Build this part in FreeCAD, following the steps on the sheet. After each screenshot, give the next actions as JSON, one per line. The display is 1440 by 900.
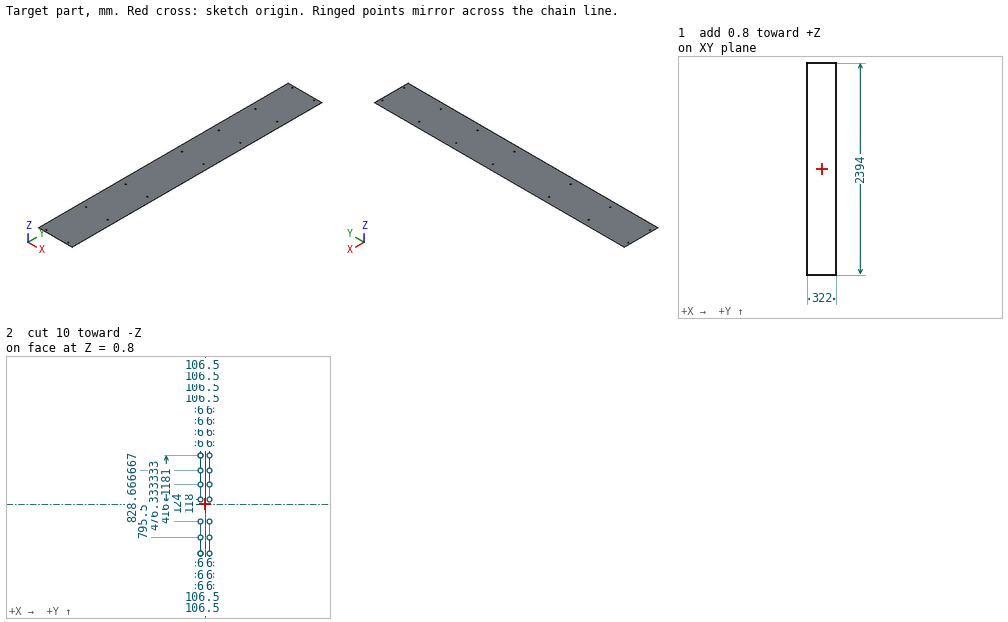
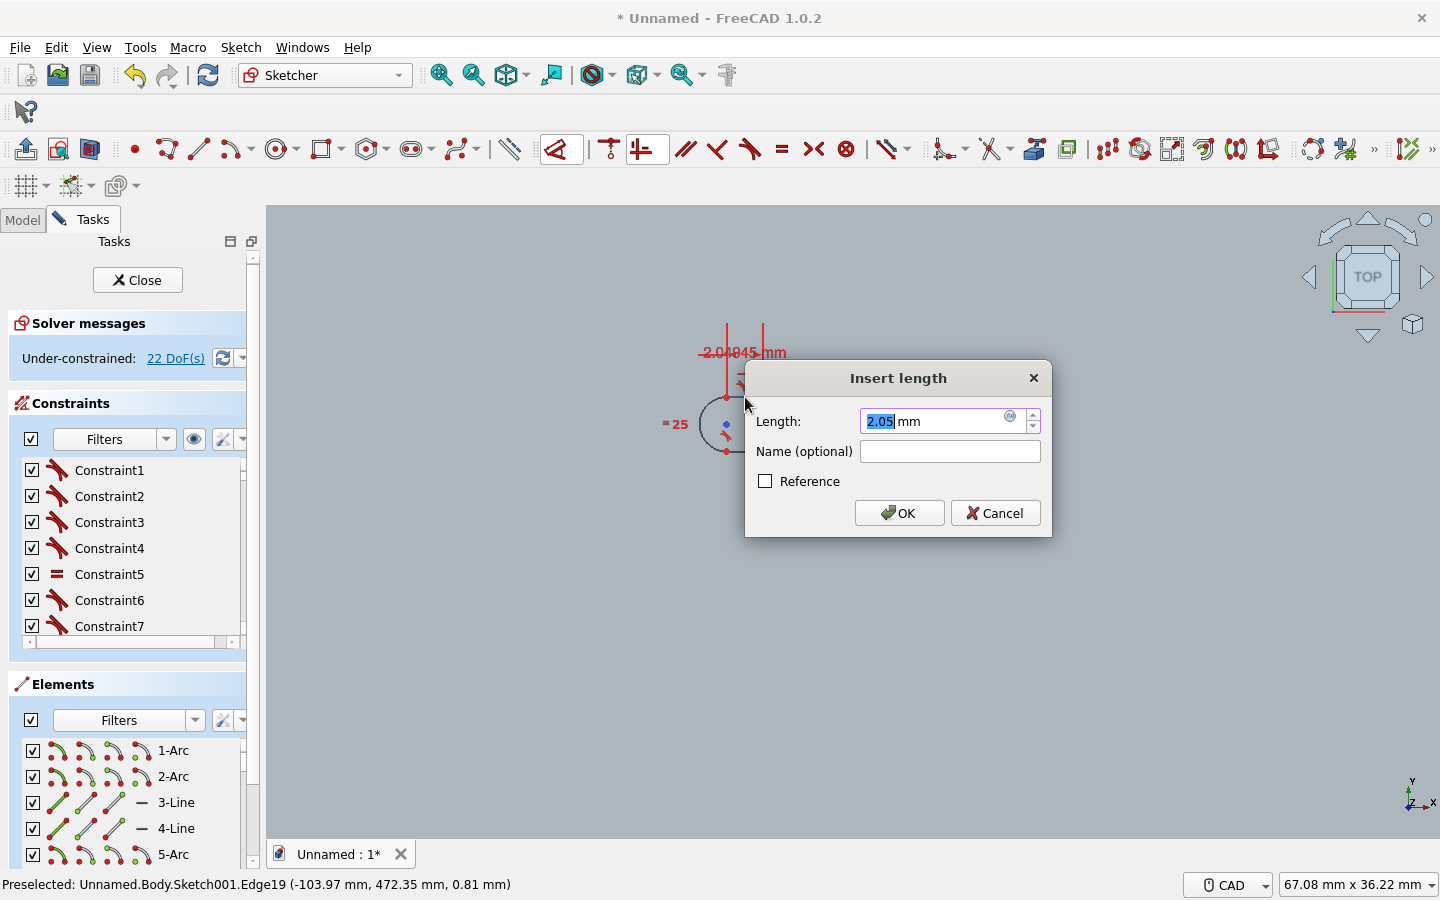
{"action": "type", "text": "6"}
{"action": "key", "text": "Return"}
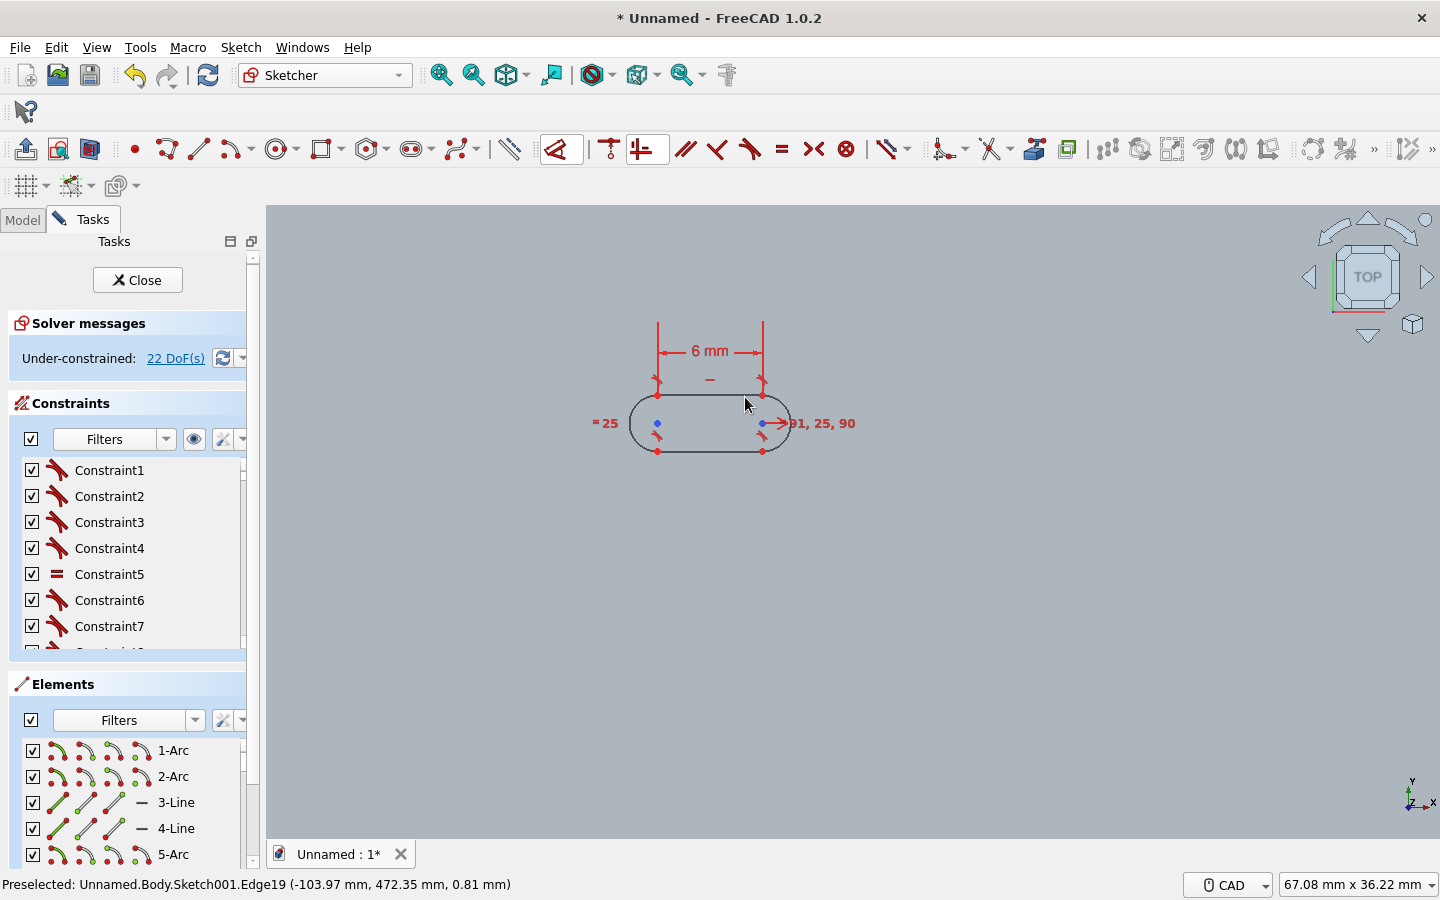
{"action": "scroll", "coordinate": [784, 522], "scroll_direction": "down", "scroll_amount": 15}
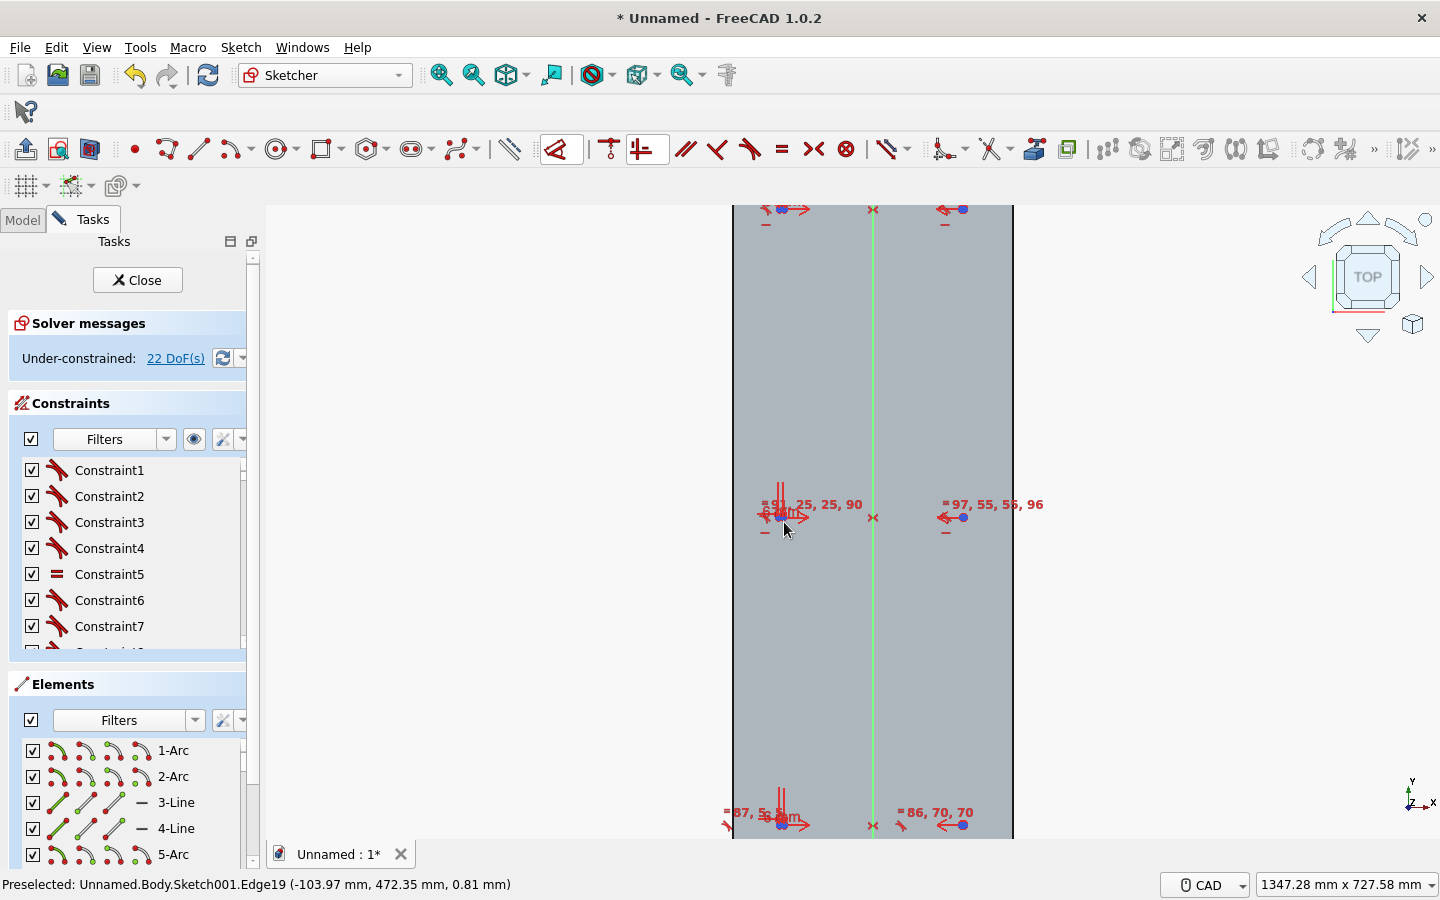
{"action": "scroll", "coordinate": [762, 419], "scroll_direction": "down", "scroll_amount": 8}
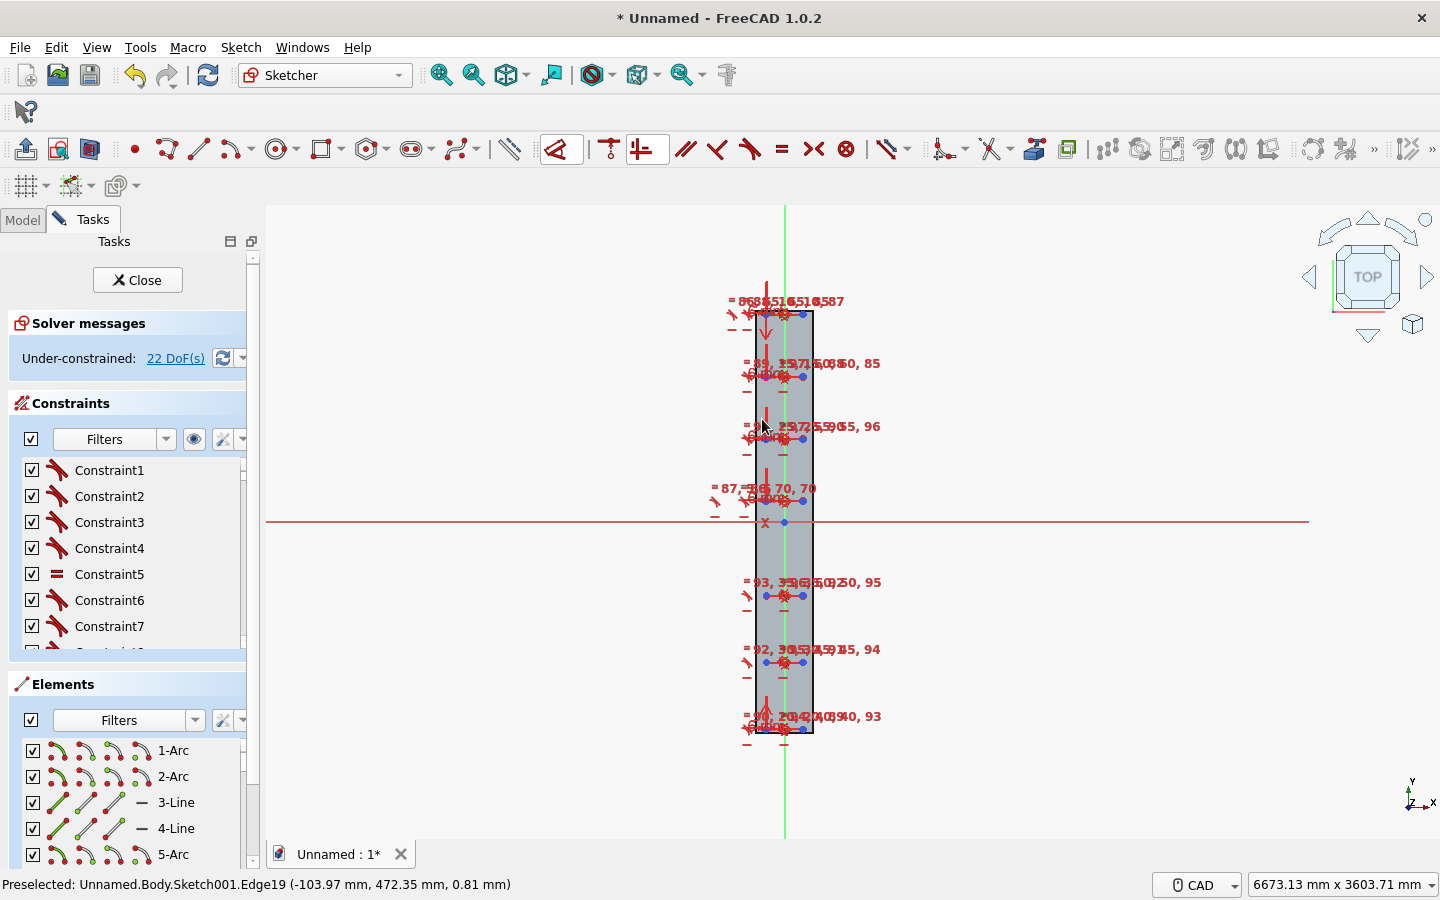
{"action": "scroll", "coordinate": [766, 662], "scroll_direction": "up", "scroll_amount": 19}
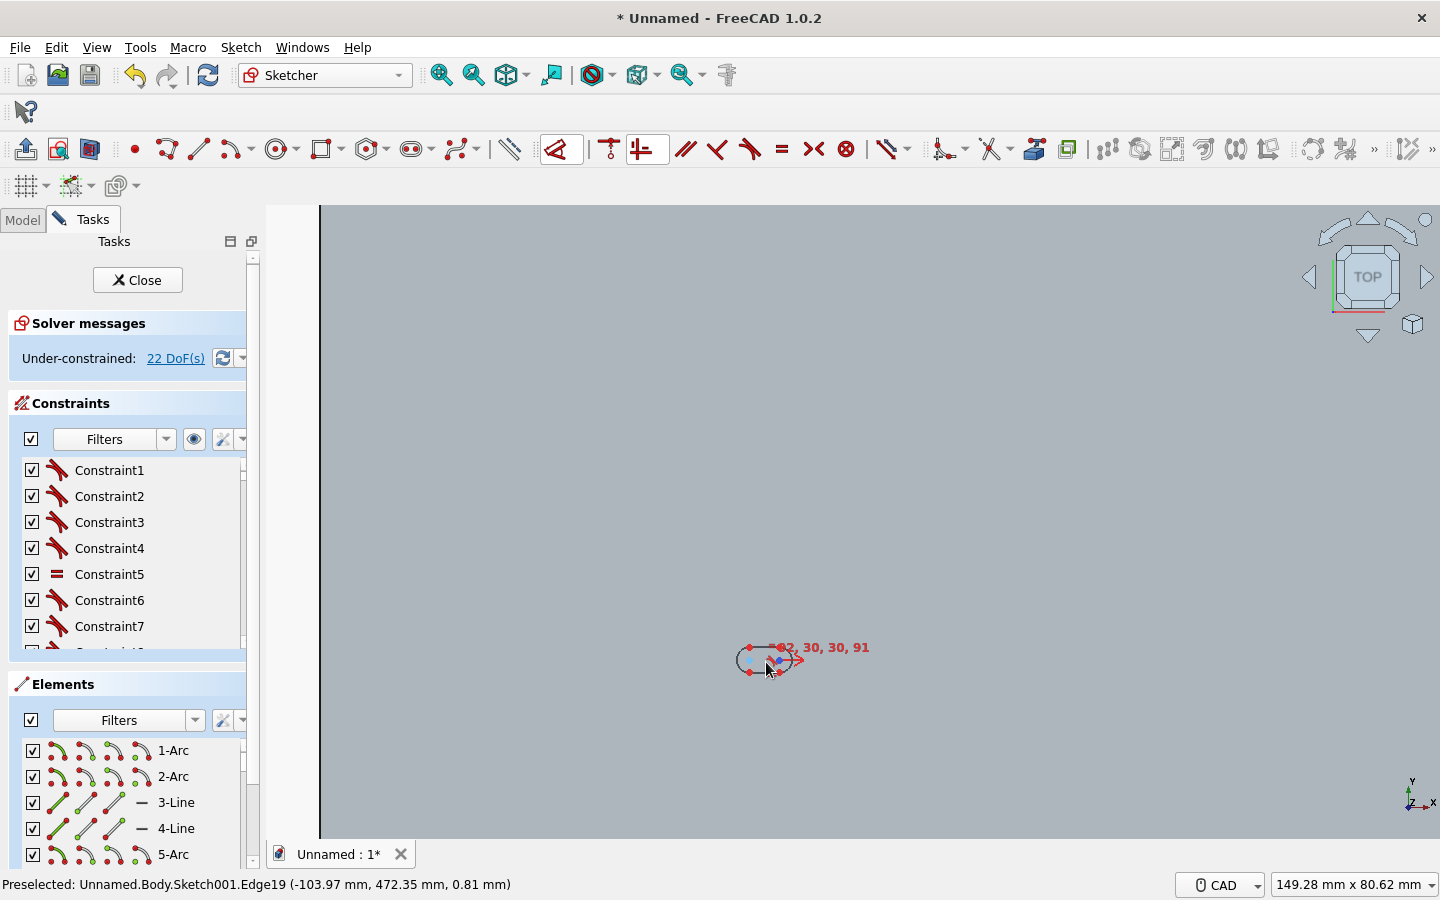
{"action": "left_click", "coordinate": [758, 647]}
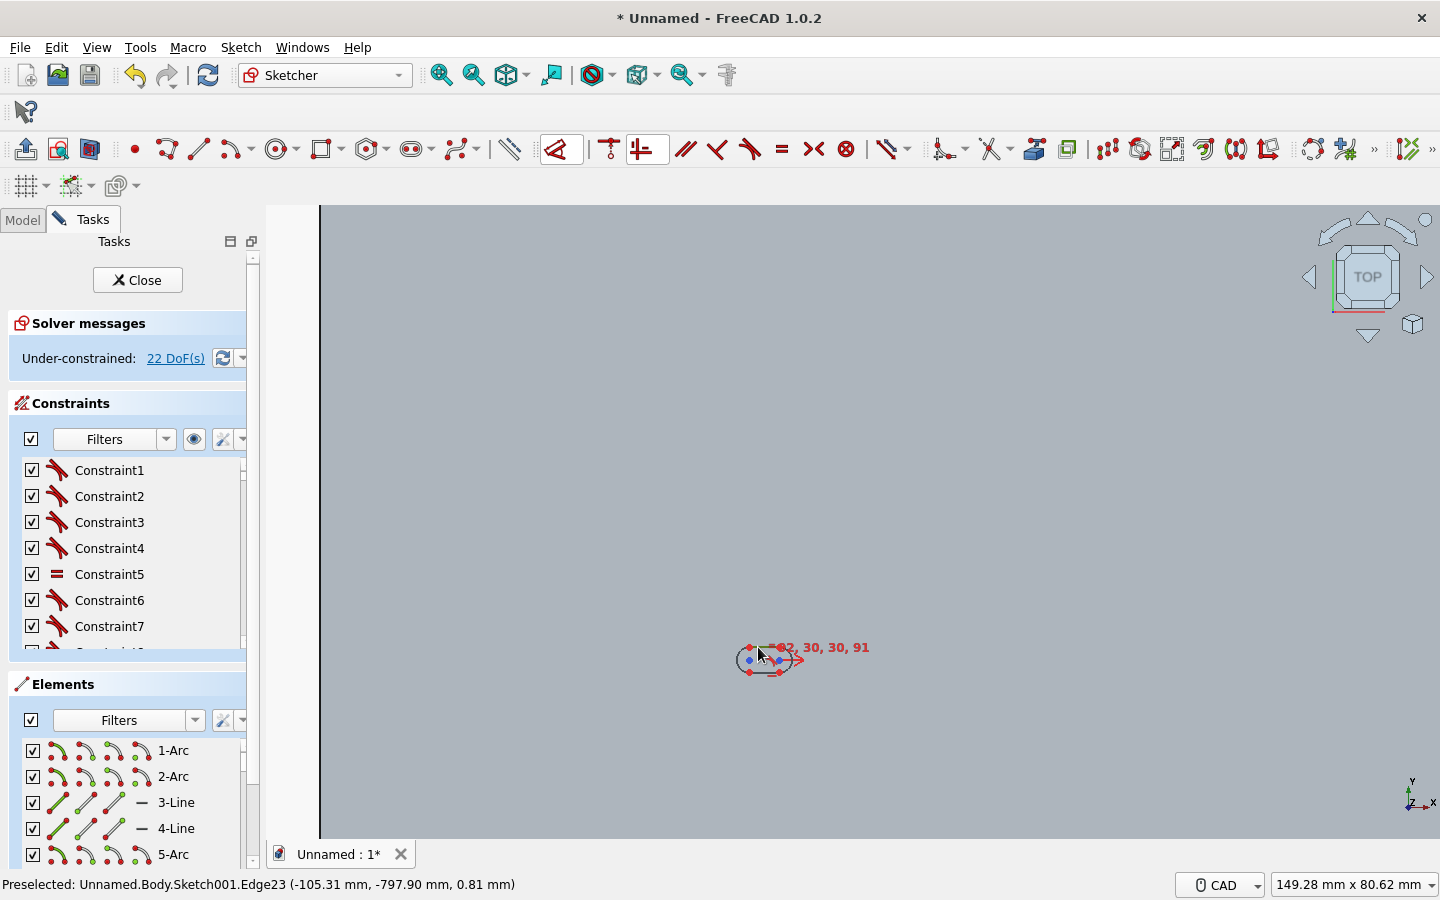
{"action": "key", "text": "l"}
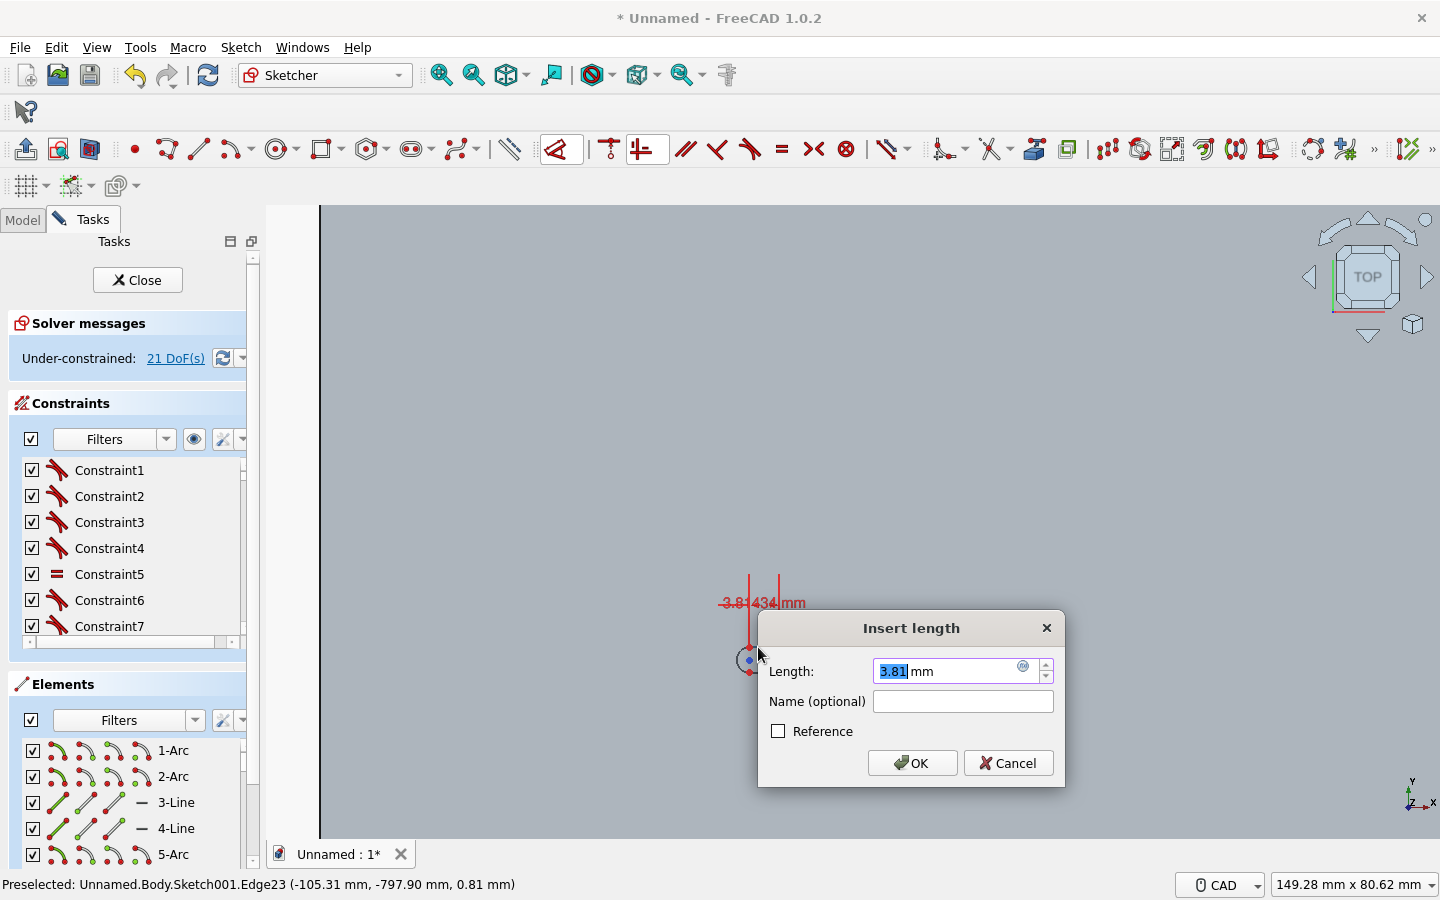
{"action": "type", "text": "6"}
{"action": "key", "text": "Return"}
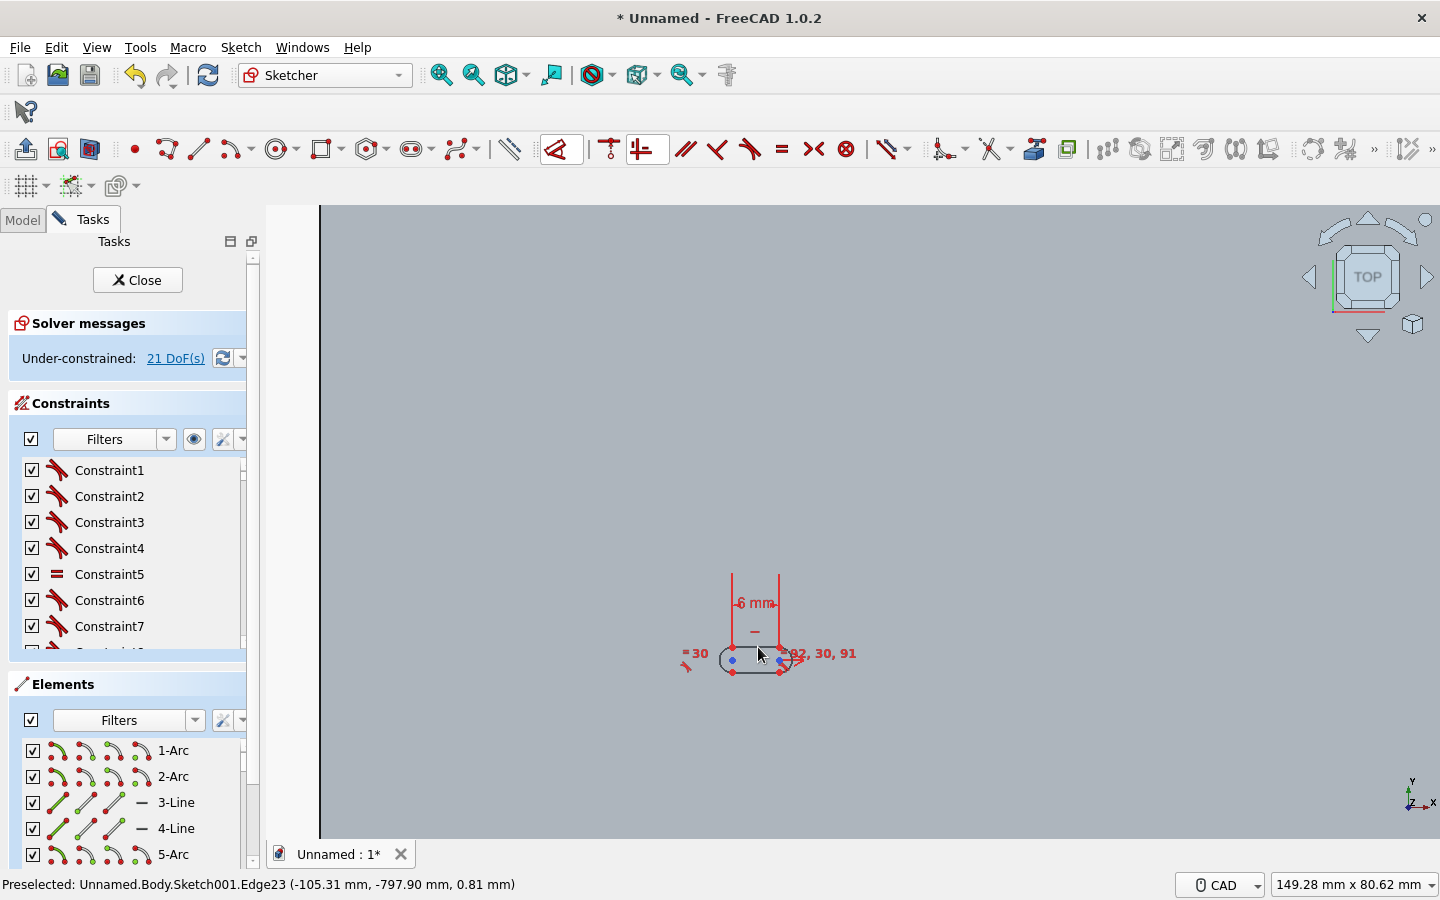
{"action": "scroll", "coordinate": [762, 695], "scroll_direction": "down", "scroll_amount": 18}